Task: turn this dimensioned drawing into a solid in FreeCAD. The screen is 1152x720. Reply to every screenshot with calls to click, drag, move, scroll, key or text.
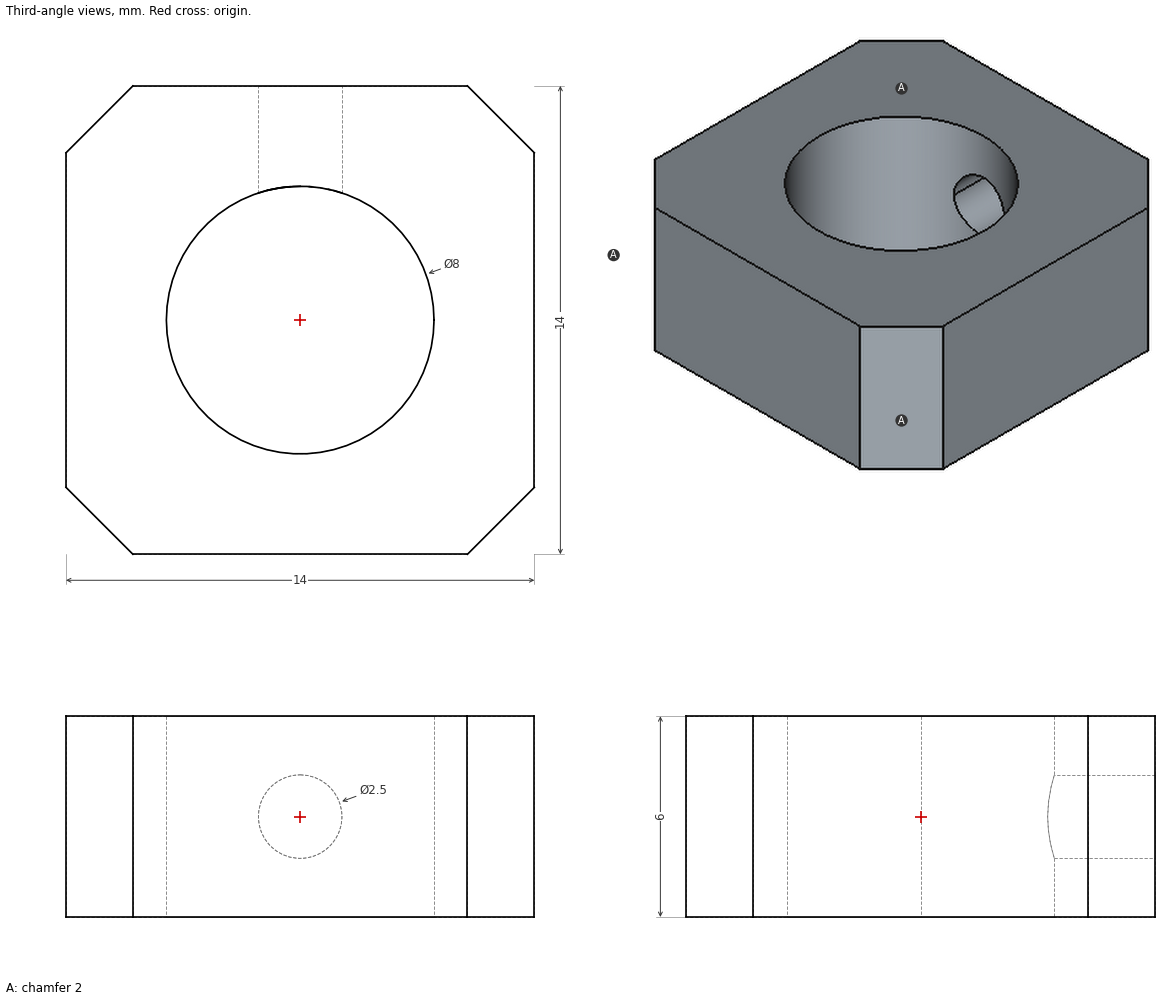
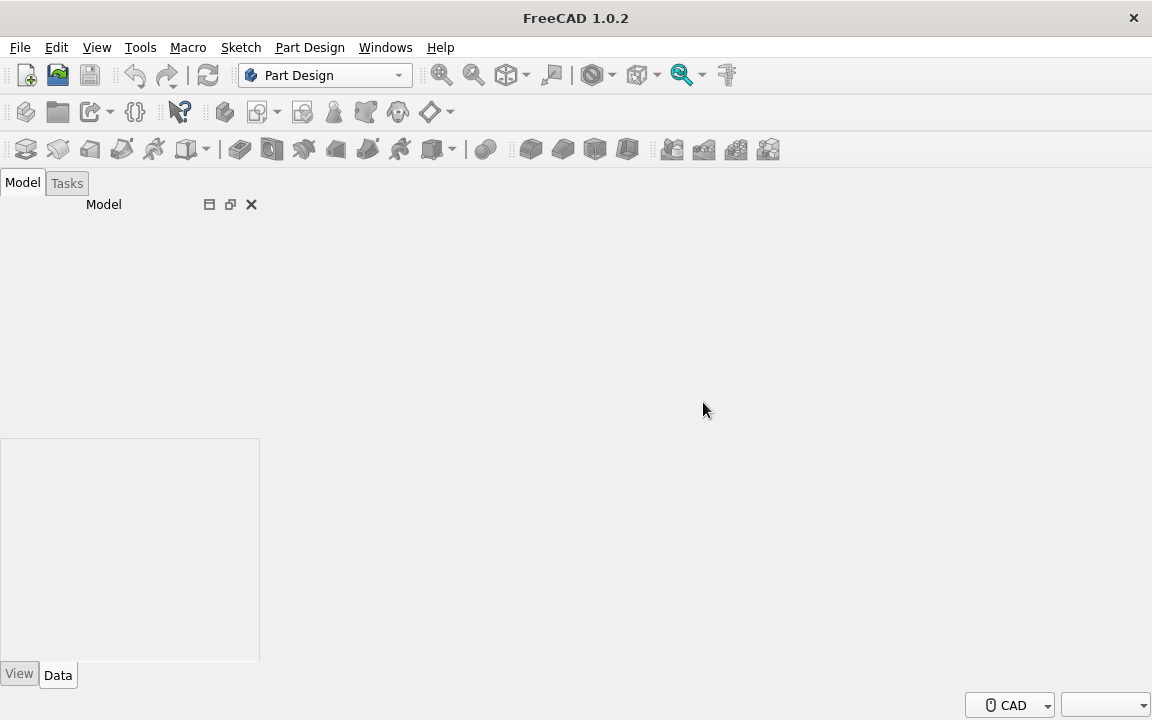
click(26, 76)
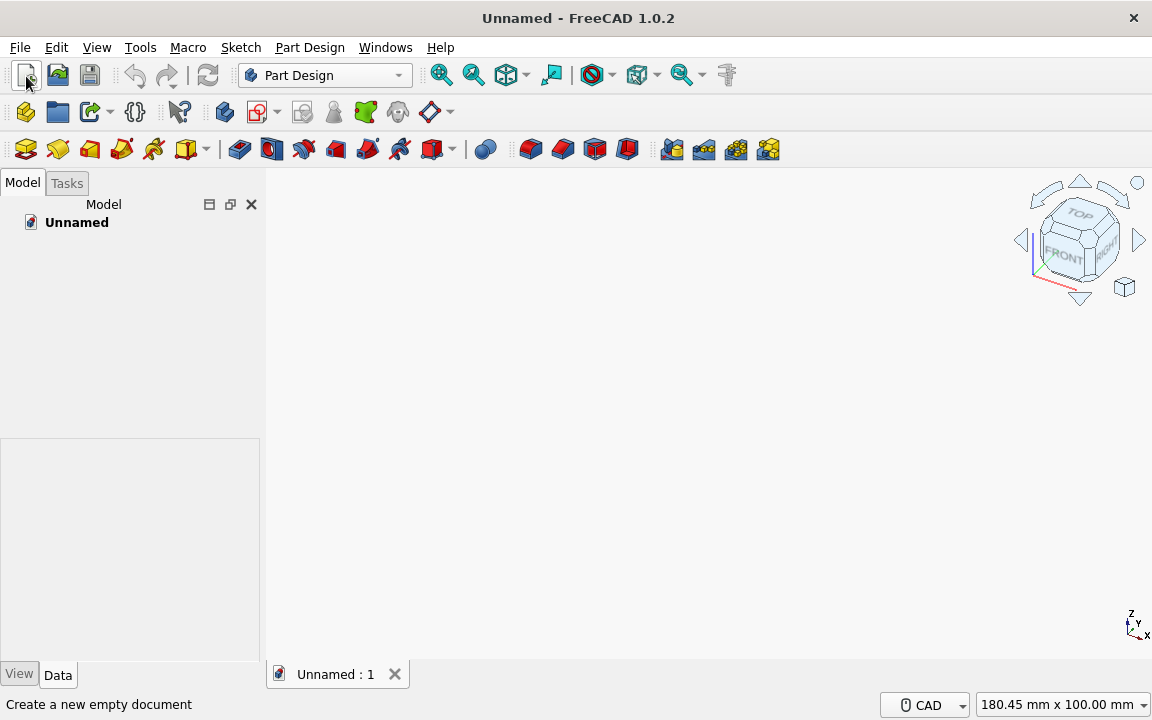
click(258, 112)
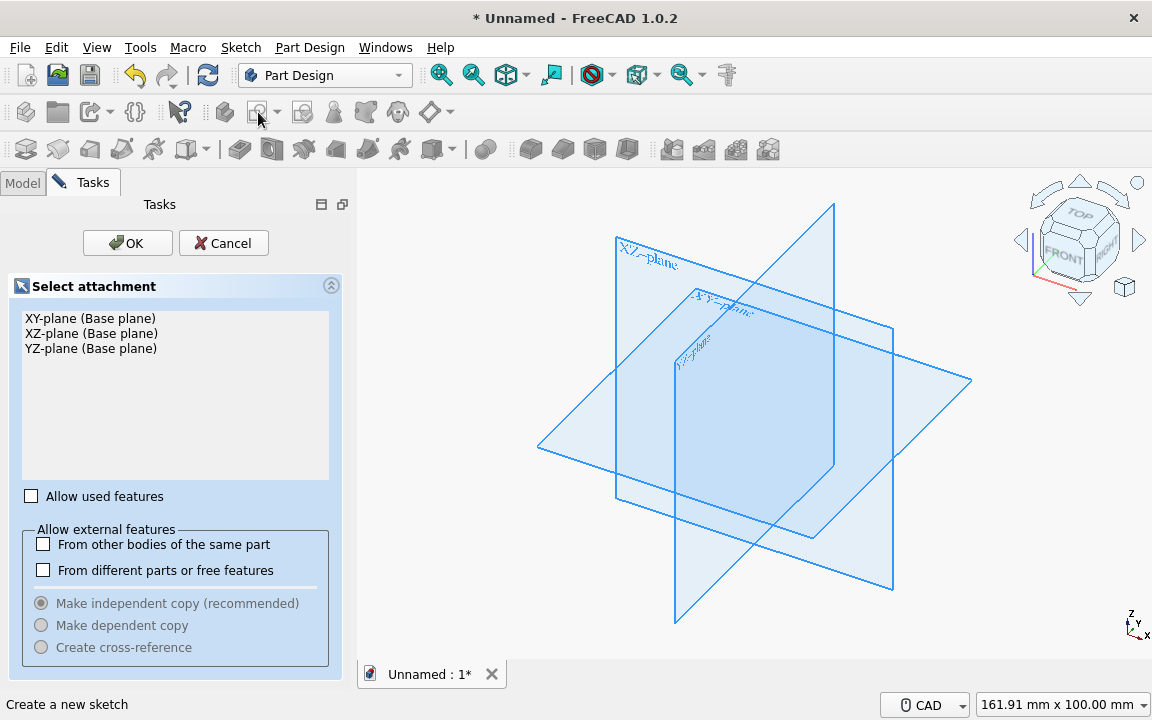
click(82, 318)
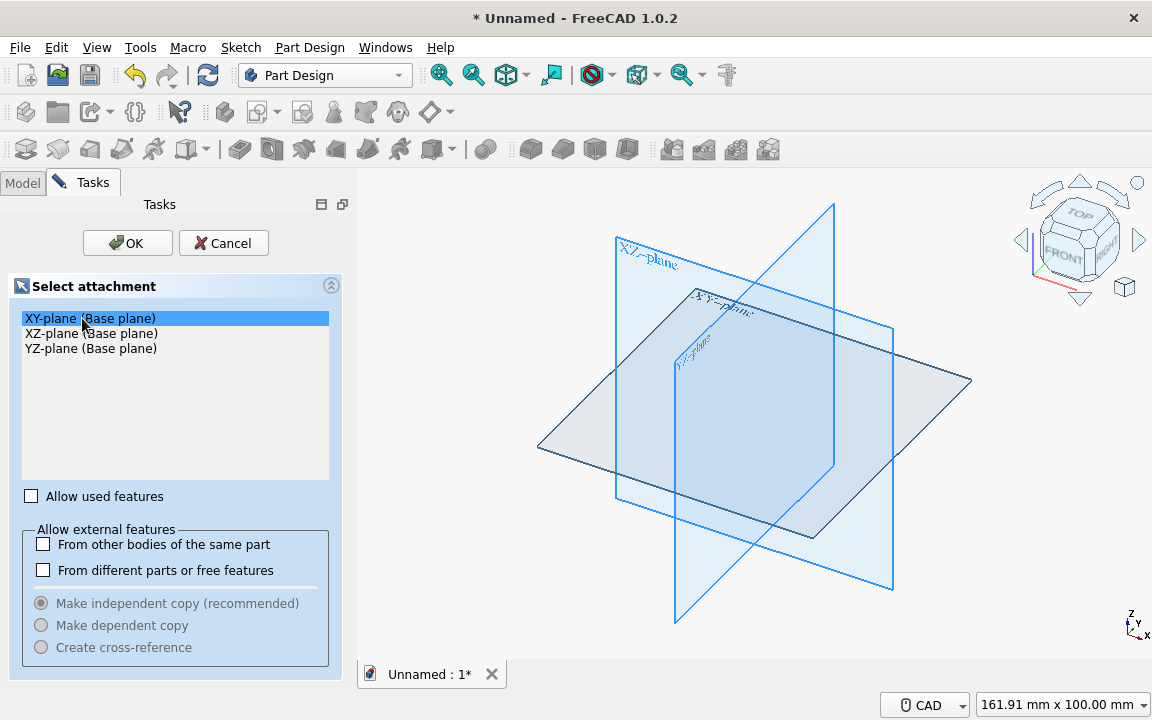
click(128, 243)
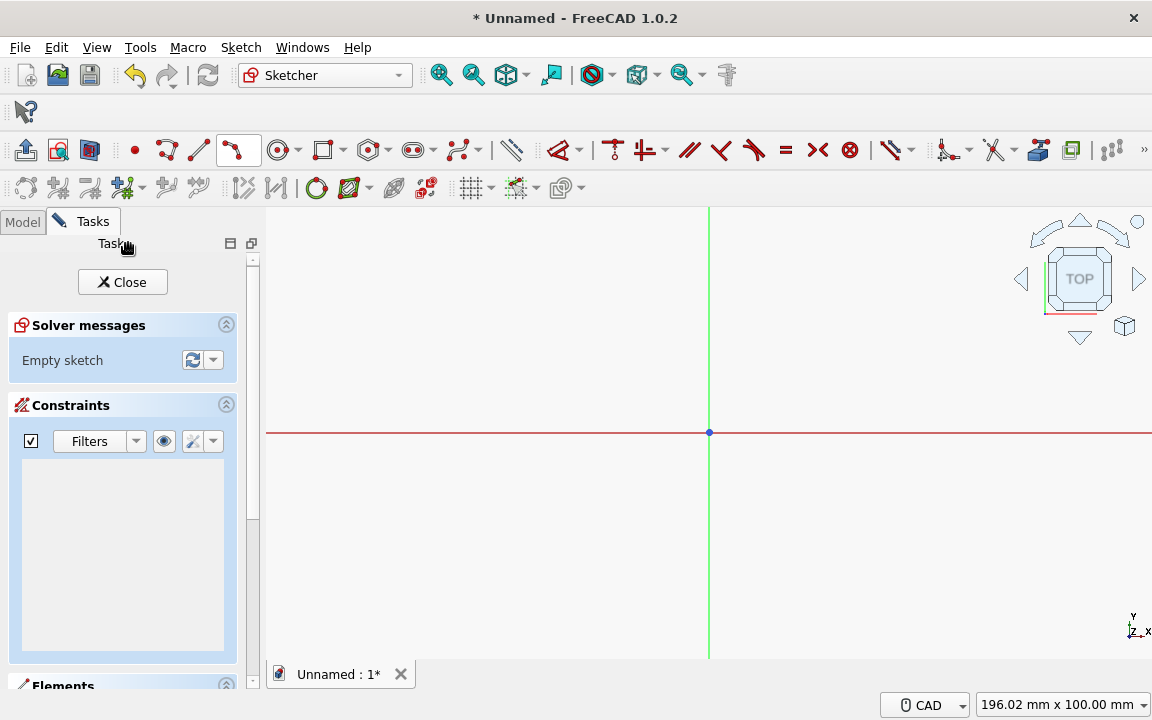
scroll(731, 433, up, 7)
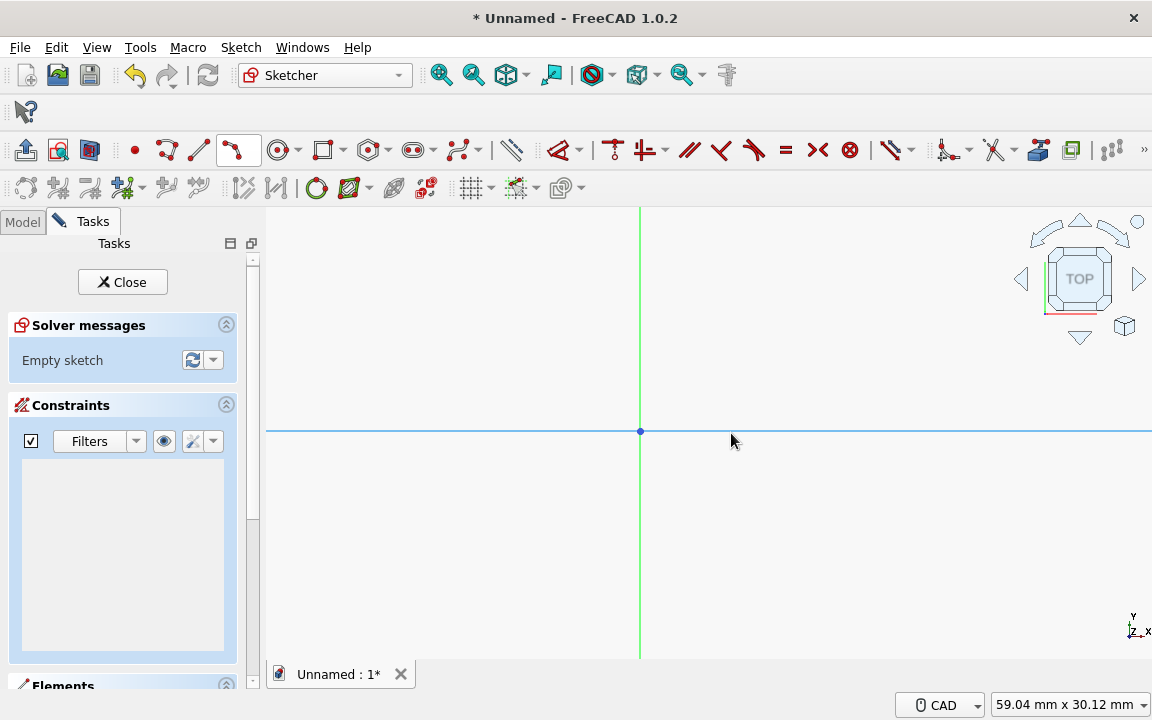
click(346, 150)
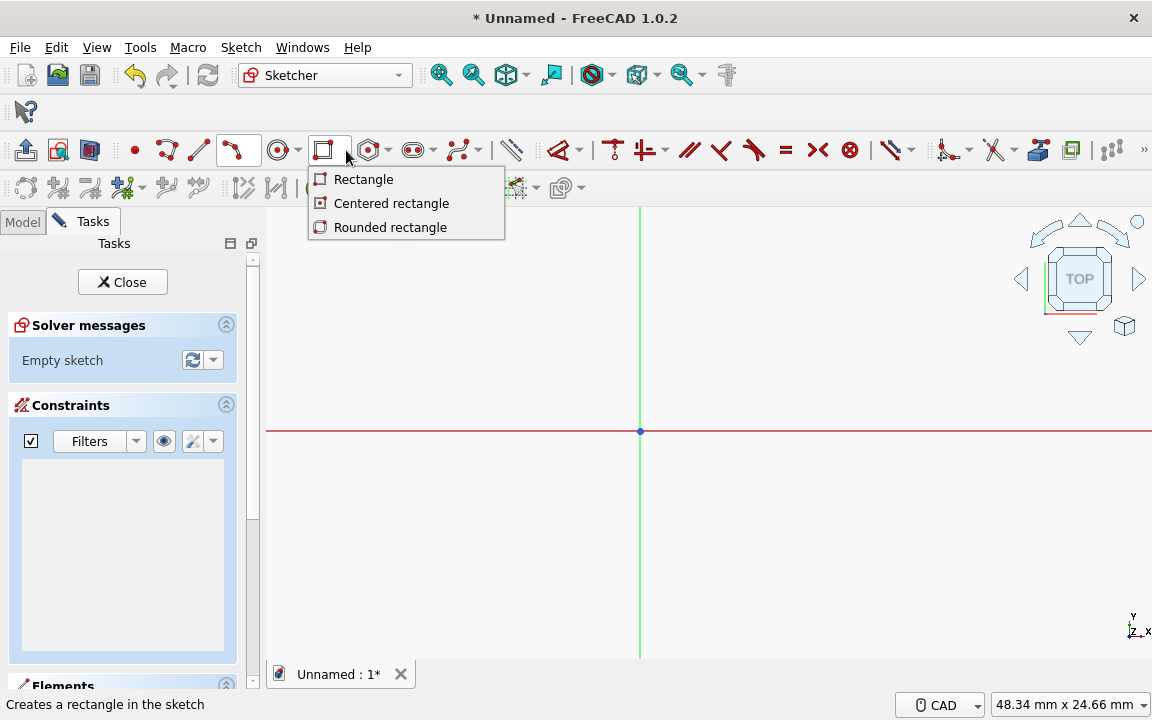
click(406, 203)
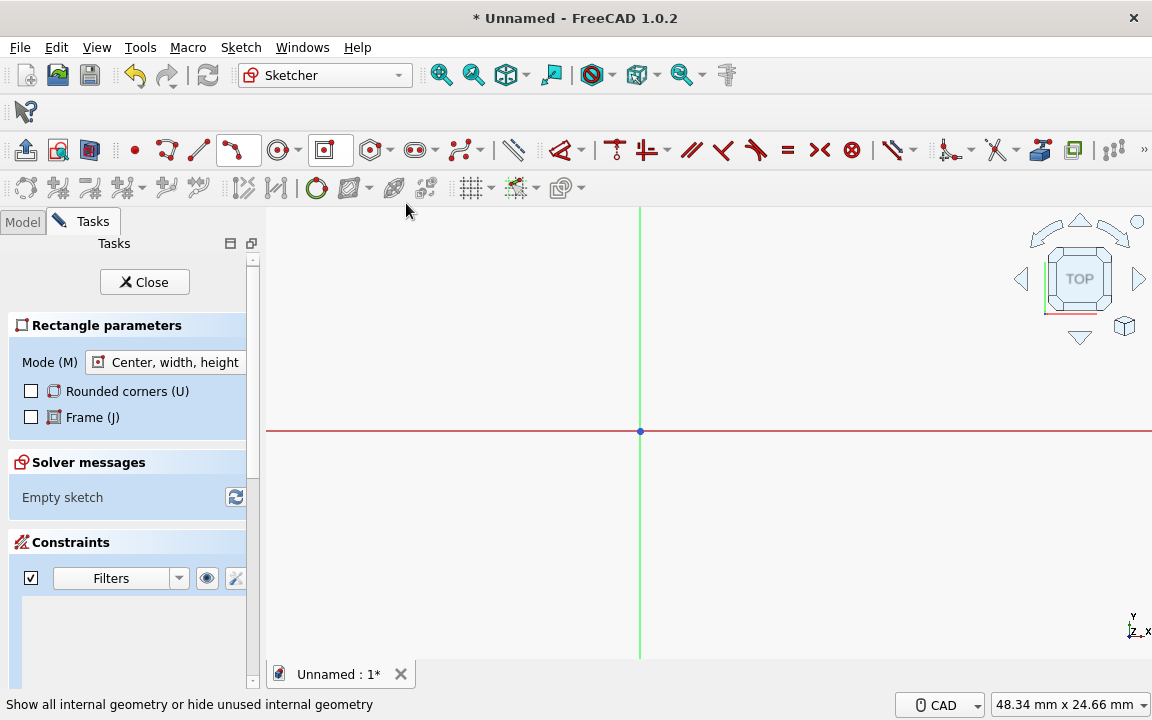
click(640, 431)
click(768, 303)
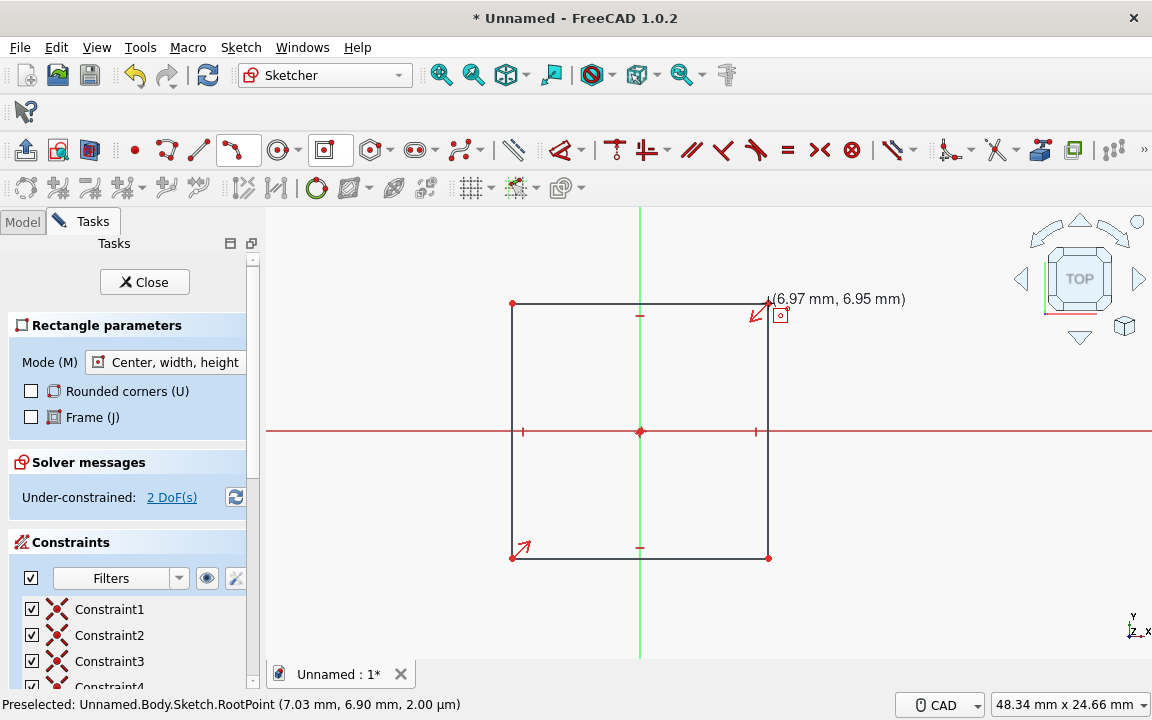
click(278, 150)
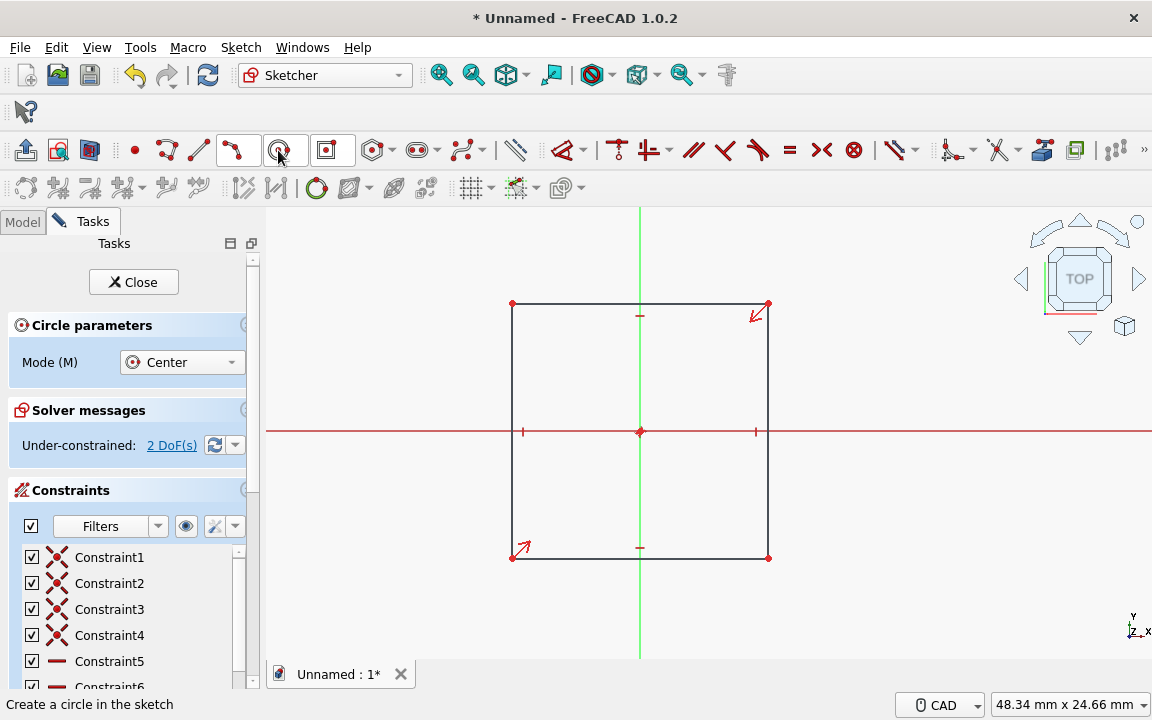
click(640, 431)
click(692, 380)
key(Escape)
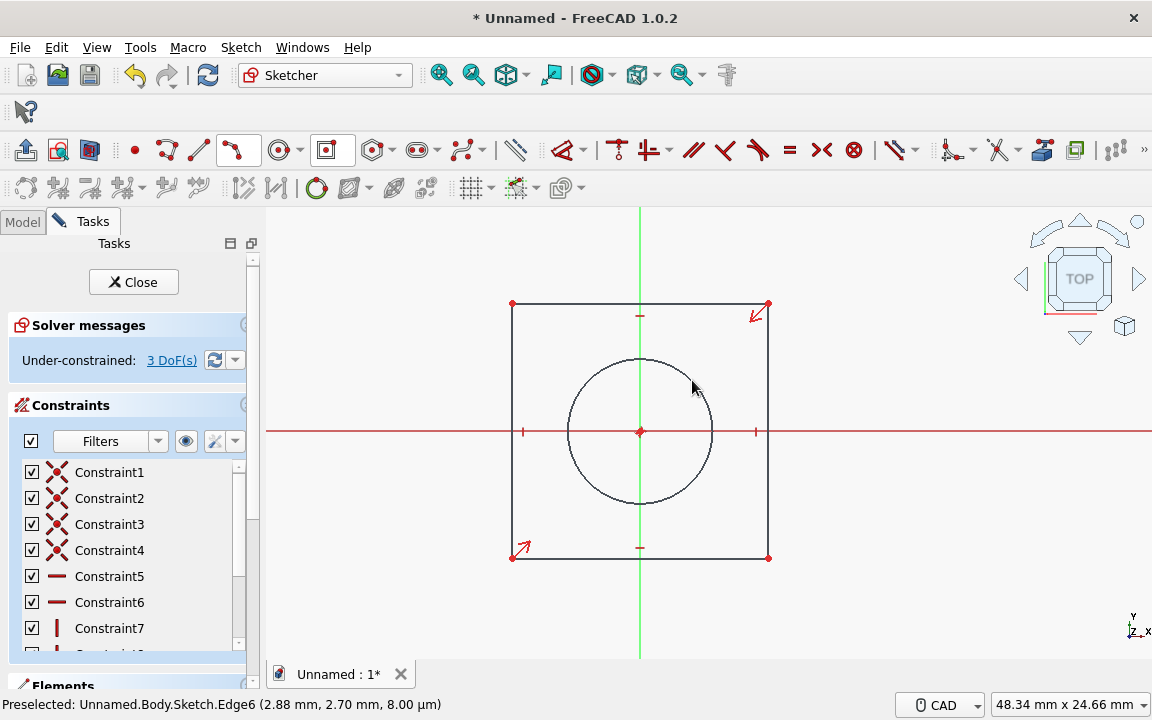
click(562, 150)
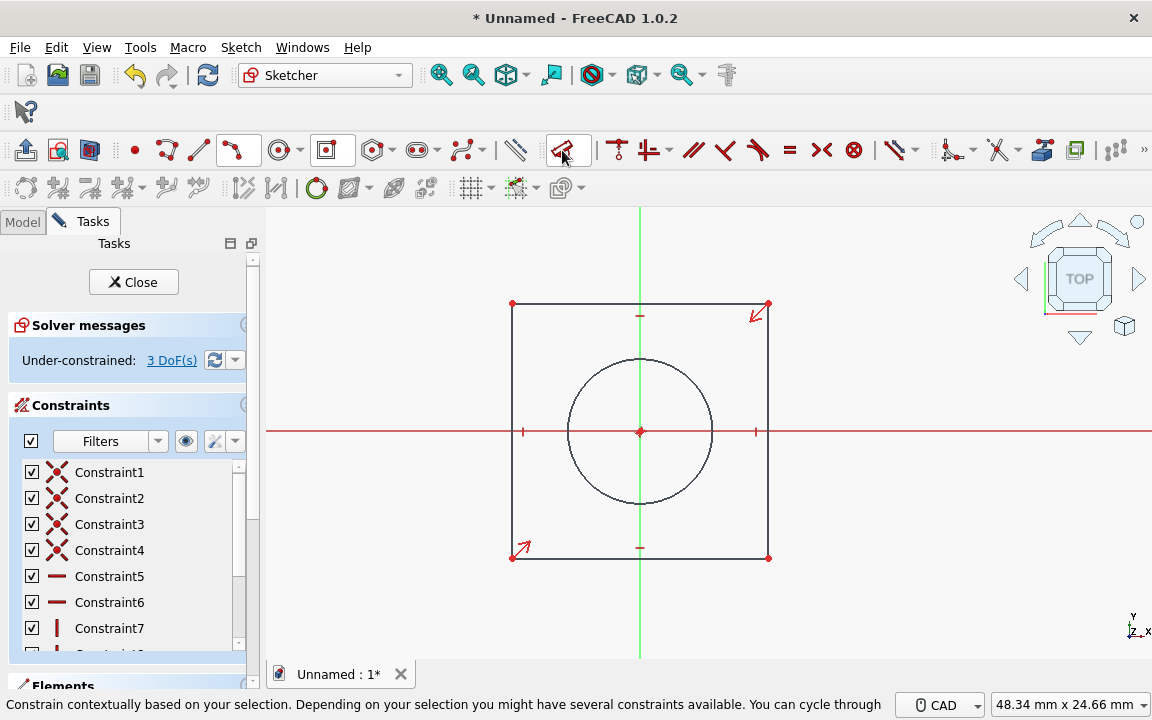
click(691, 380)
click(713, 357)